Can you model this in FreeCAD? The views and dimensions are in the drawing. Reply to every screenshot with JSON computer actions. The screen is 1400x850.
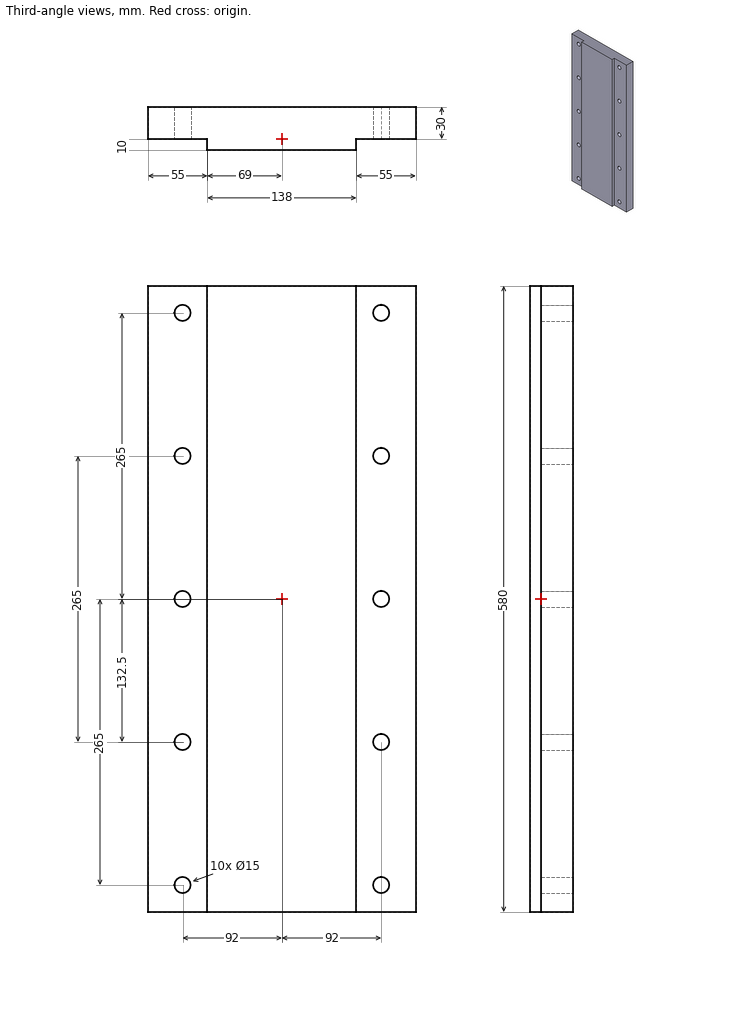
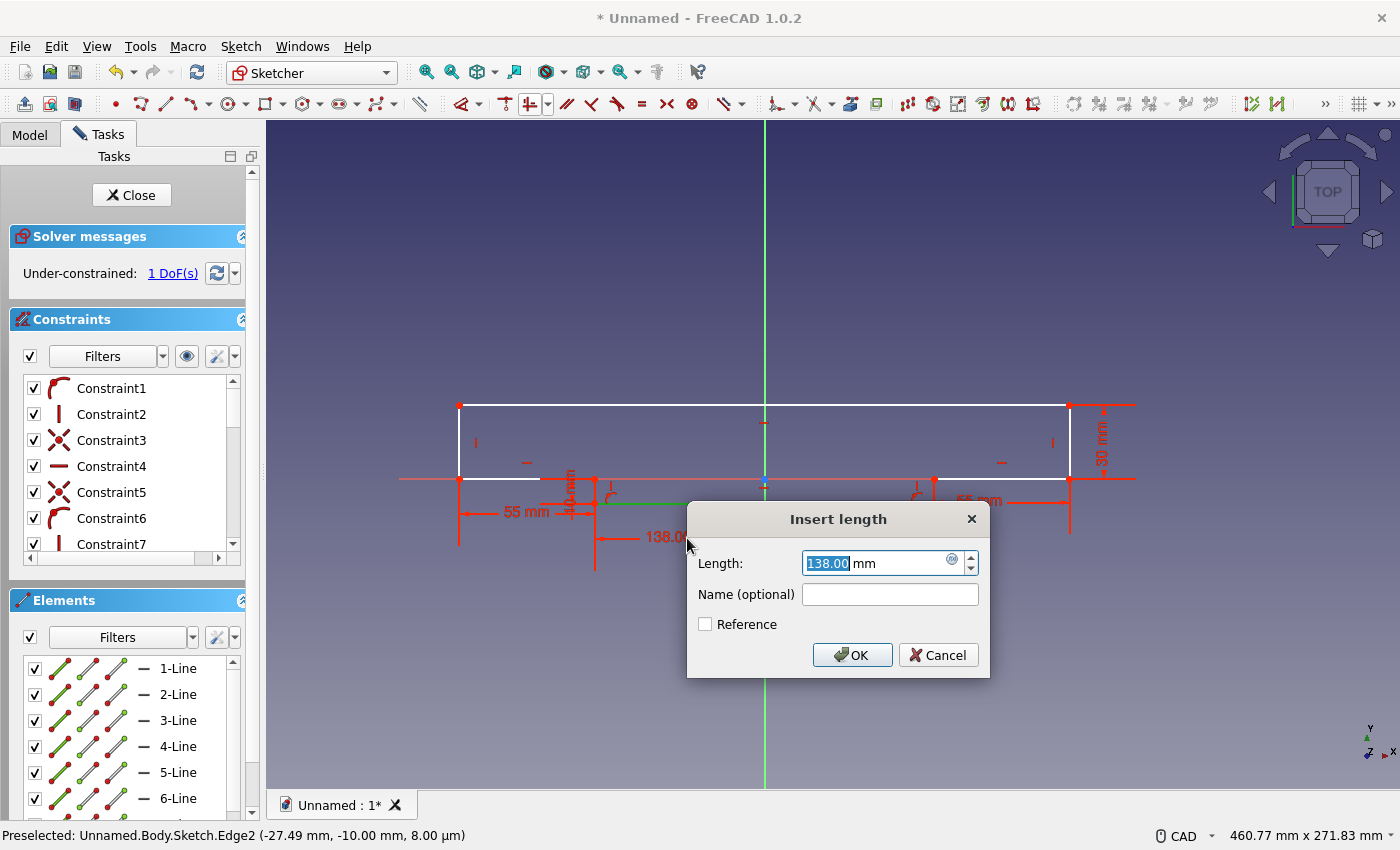
{"action": "type", "text": "138"}
{"action": "key", "text": "Return"}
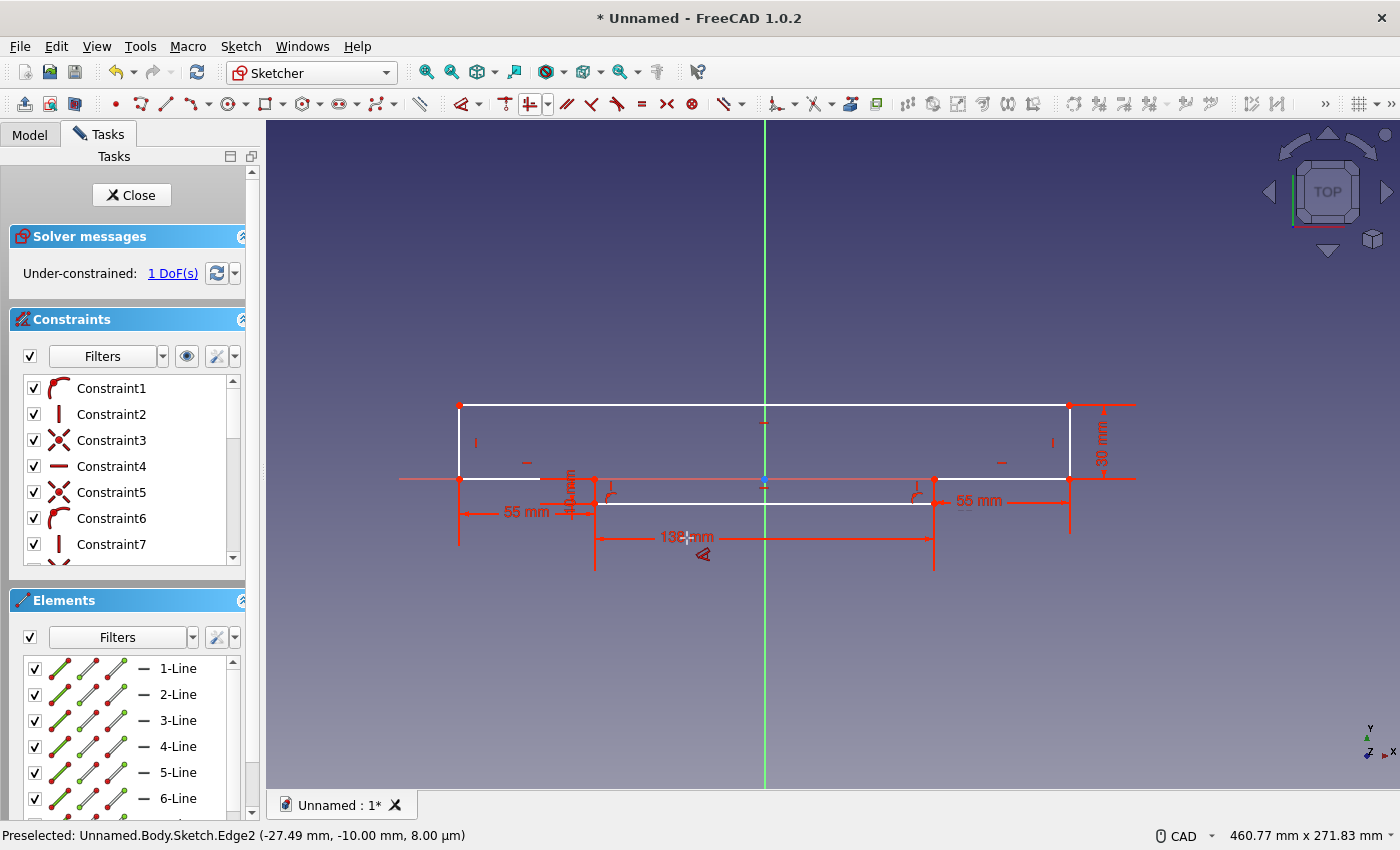
{"action": "left_click", "coordinate": [595, 479]}
{"action": "left_click", "coordinate": [680, 445]}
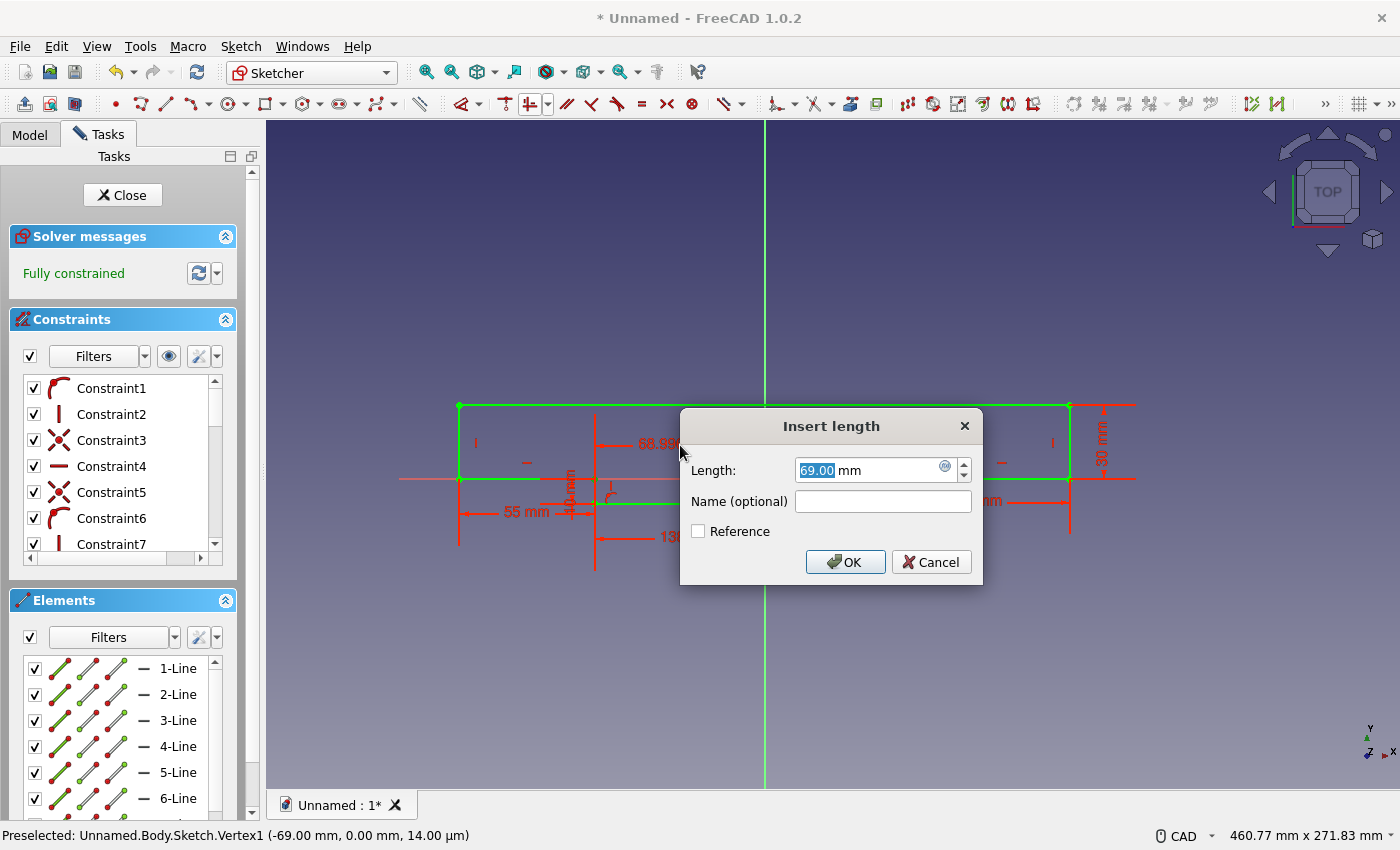
{"action": "type", "text": "69"}
{"action": "key", "text": "Return"}
{"action": "key", "text": "Escape"}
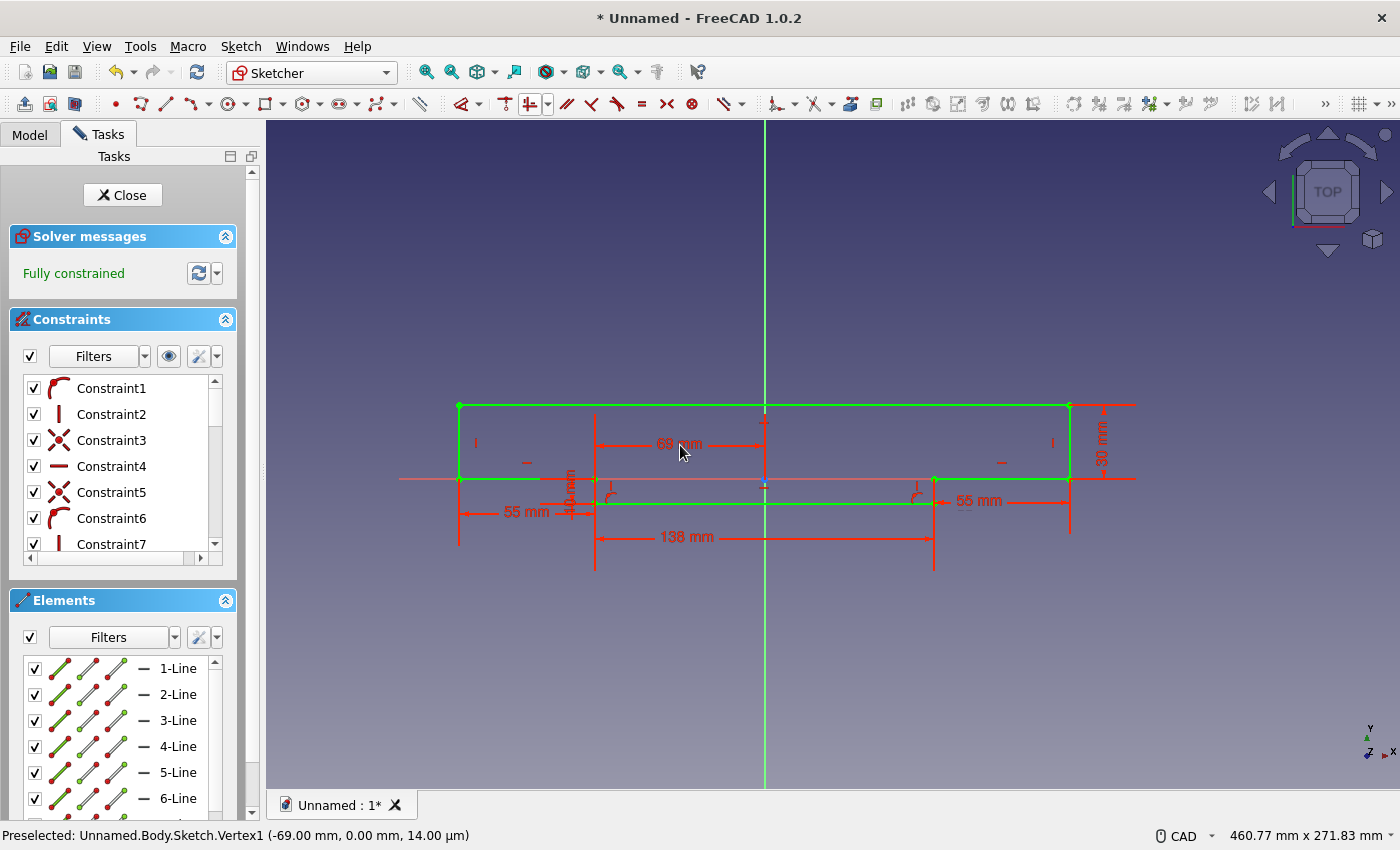
{"action": "left_click", "coordinate": [123, 195]}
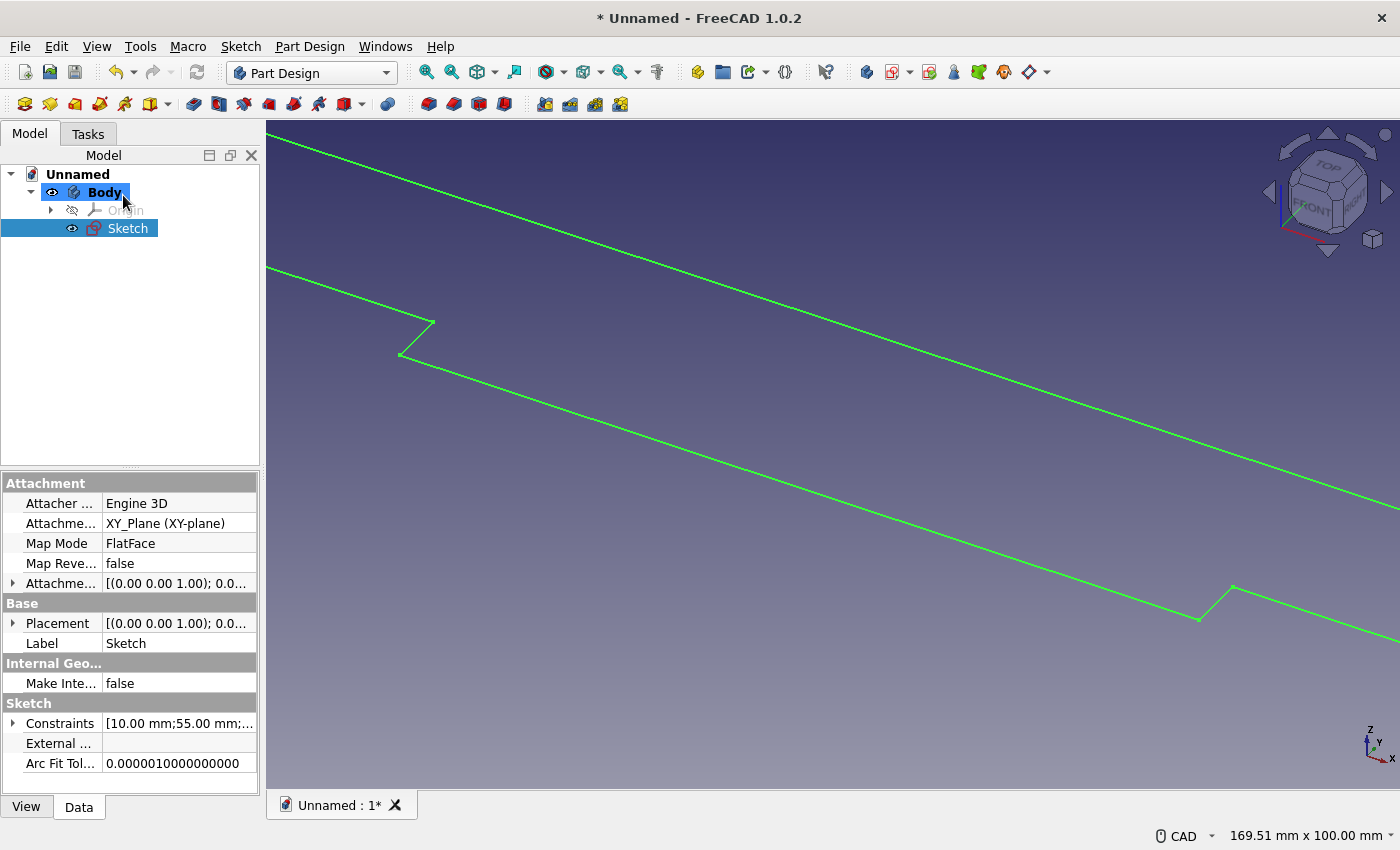
{"action": "left_click", "coordinate": [25, 104]}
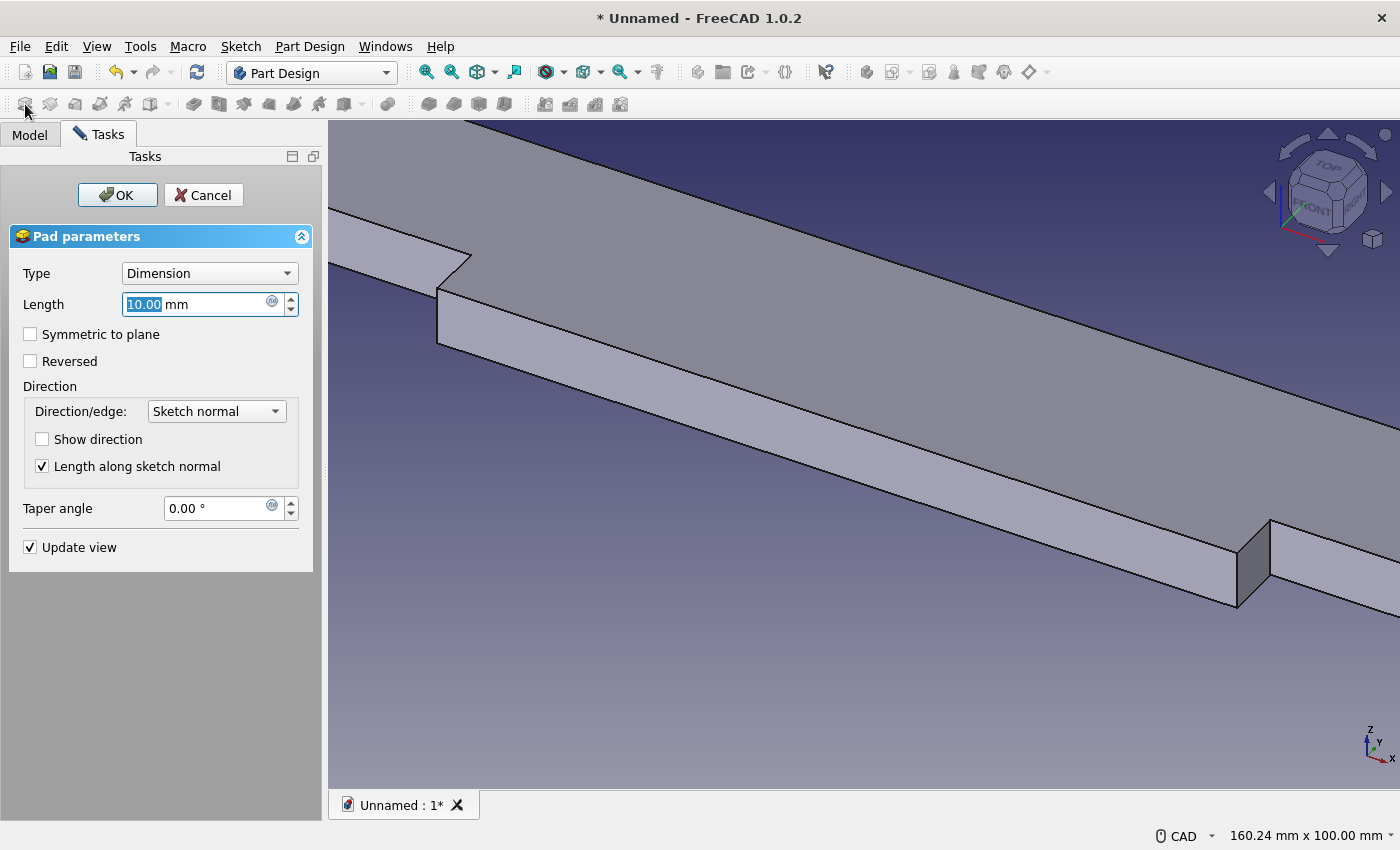
{"action": "type", "text": "580"}
{"action": "key", "text": "Tab"}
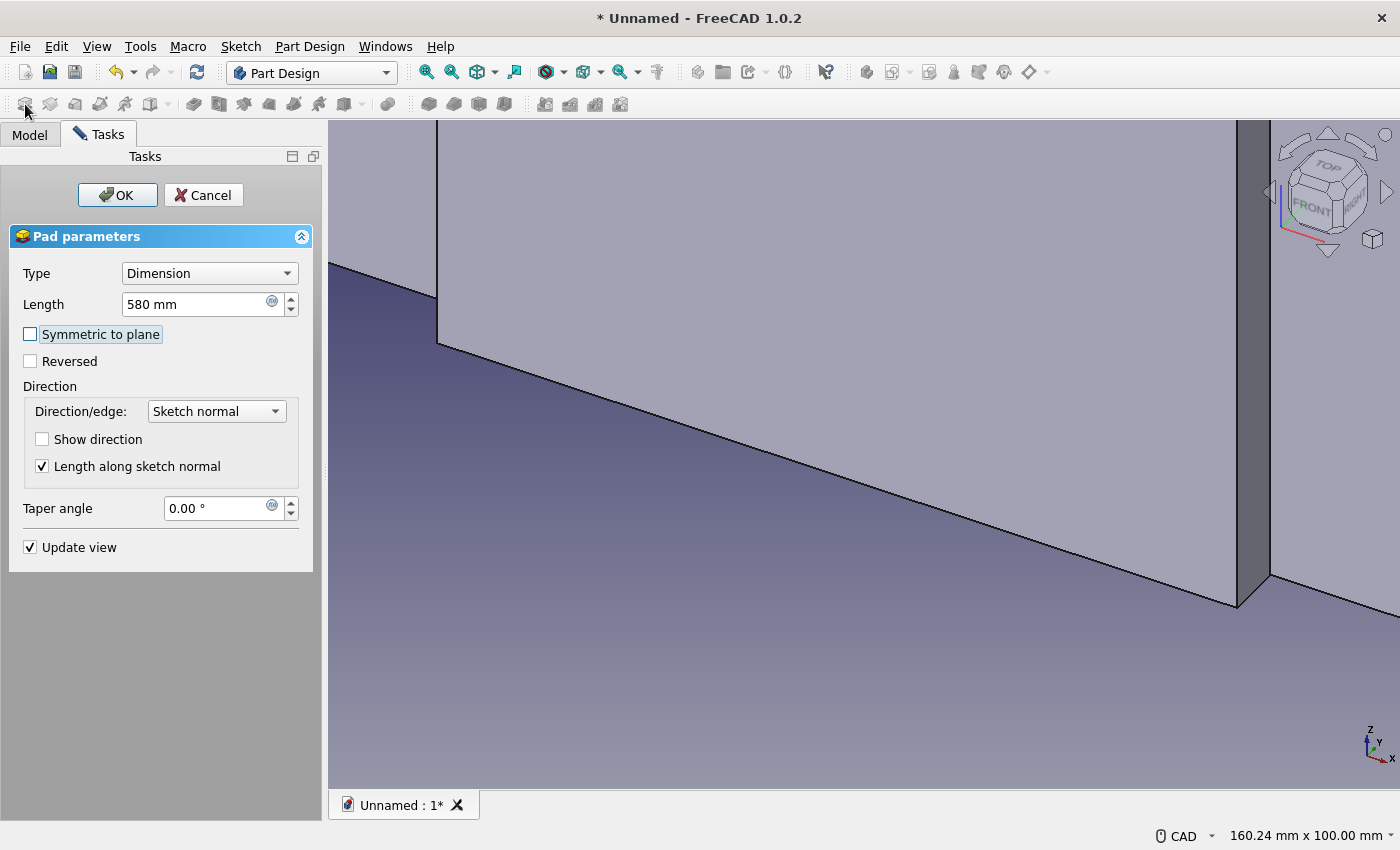
{"action": "left_click", "coordinate": [31, 334]}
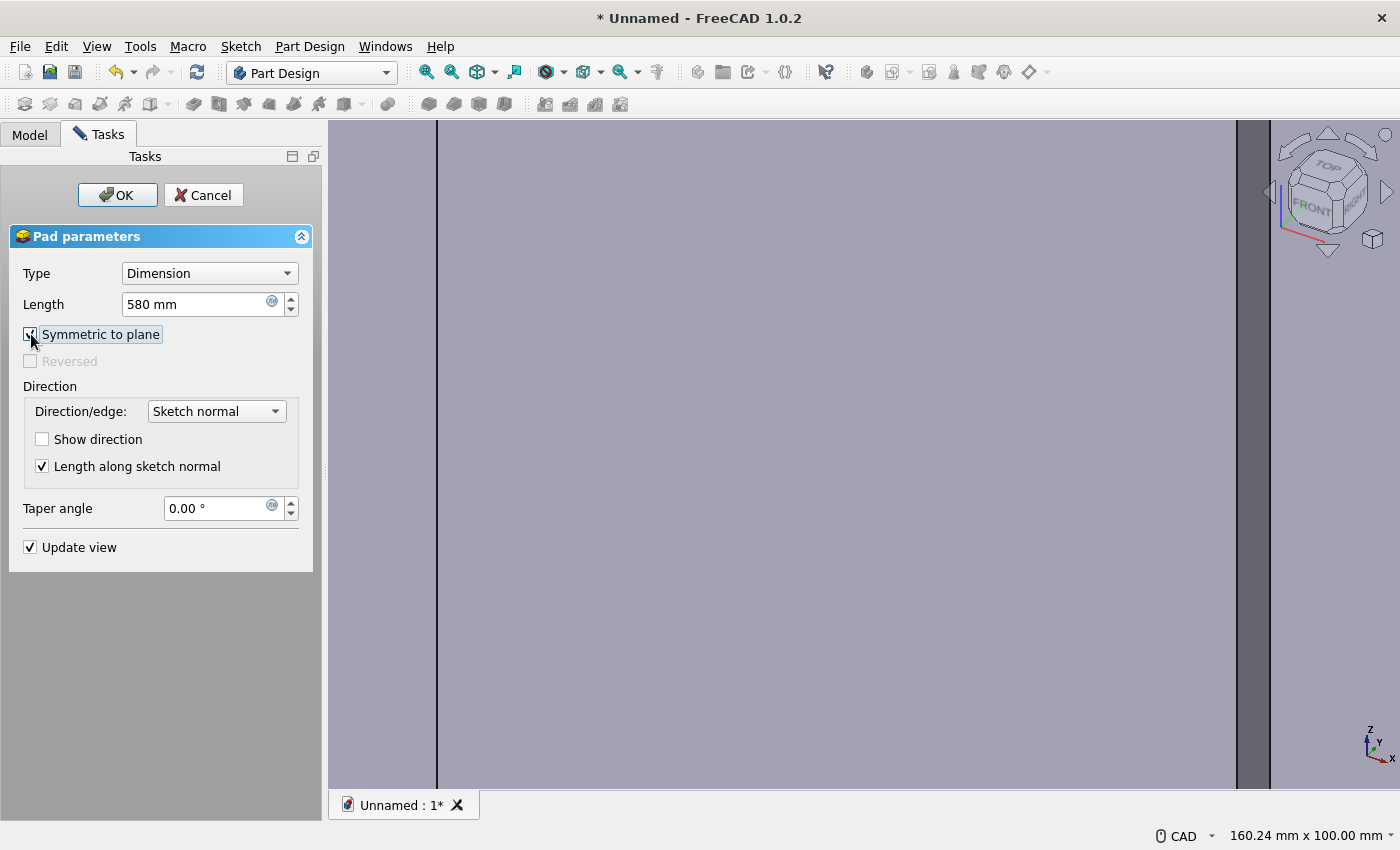
{"action": "left_click", "coordinate": [118, 195]}